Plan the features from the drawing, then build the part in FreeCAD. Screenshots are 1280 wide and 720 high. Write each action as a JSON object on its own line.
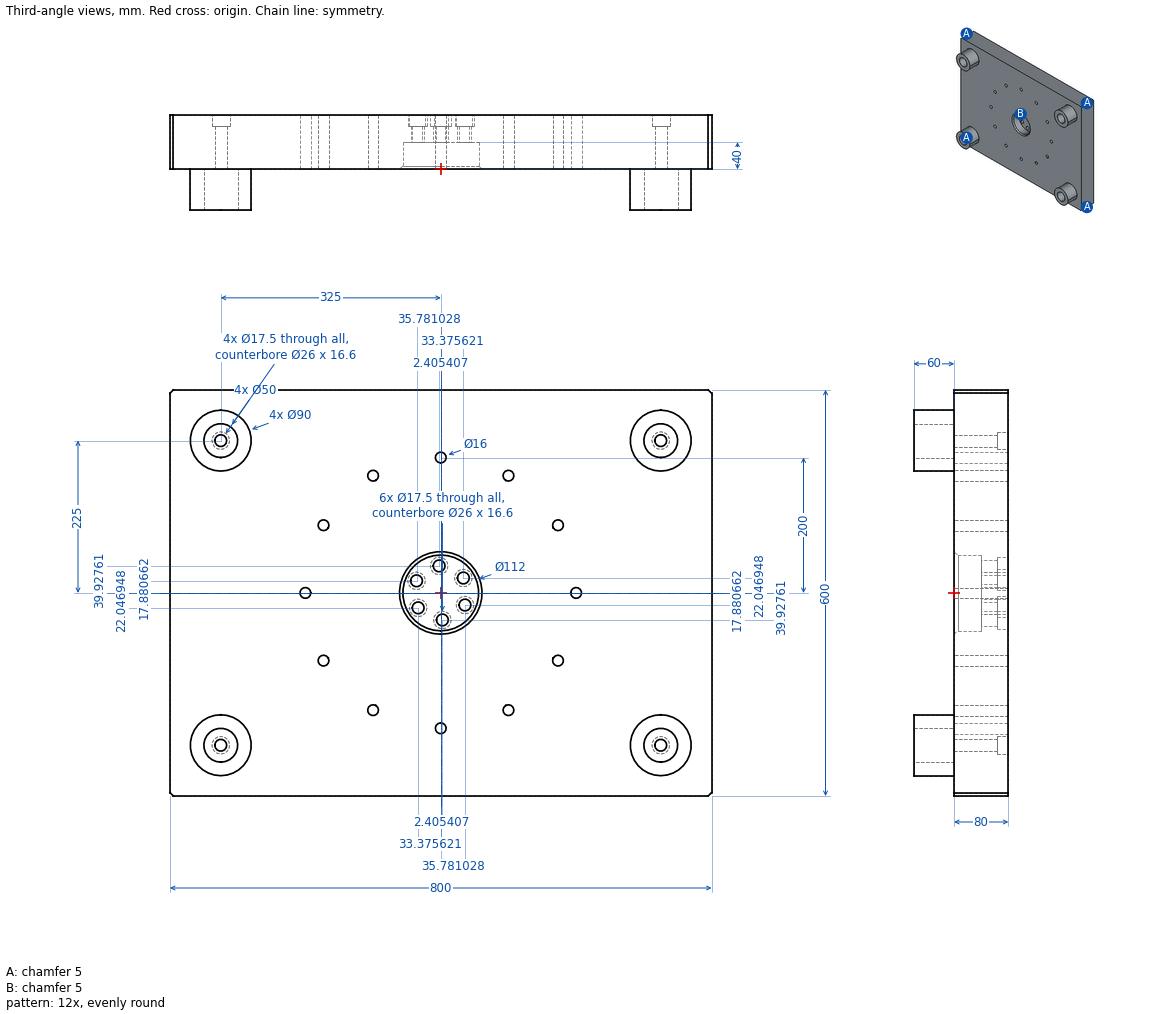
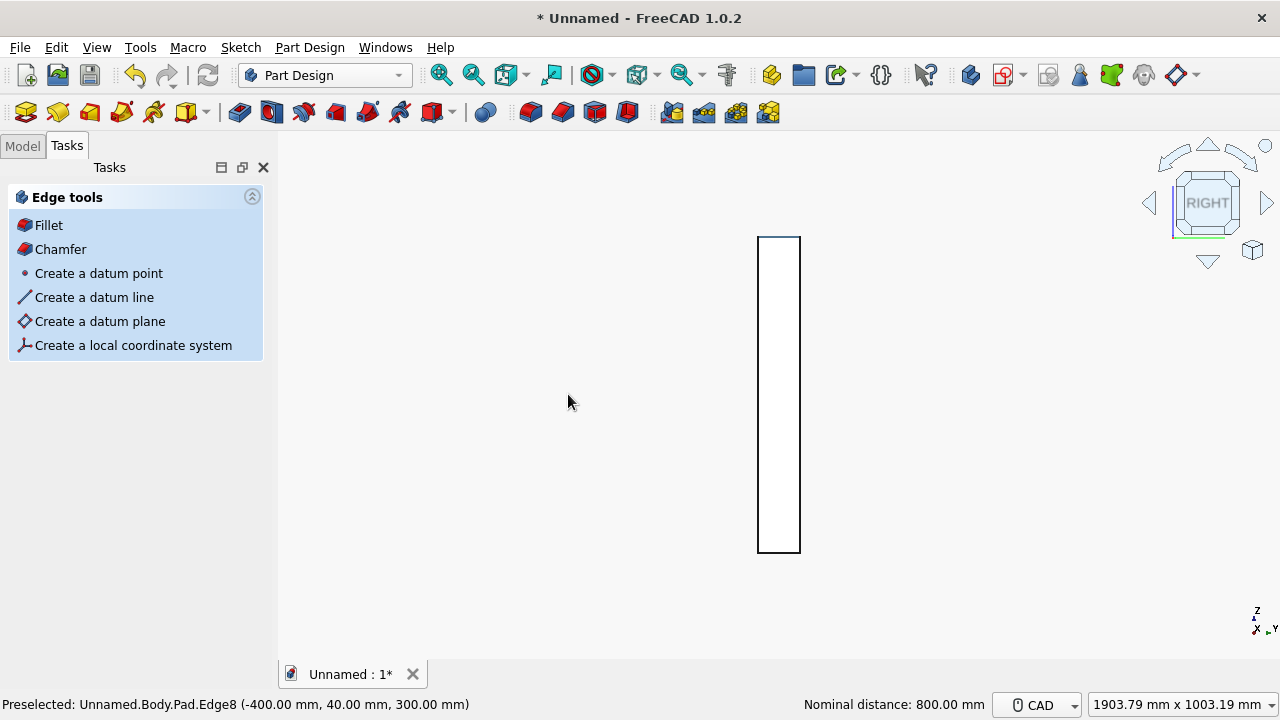
{"action": "left_click", "coordinate": [779, 552], "text": "ctrl"}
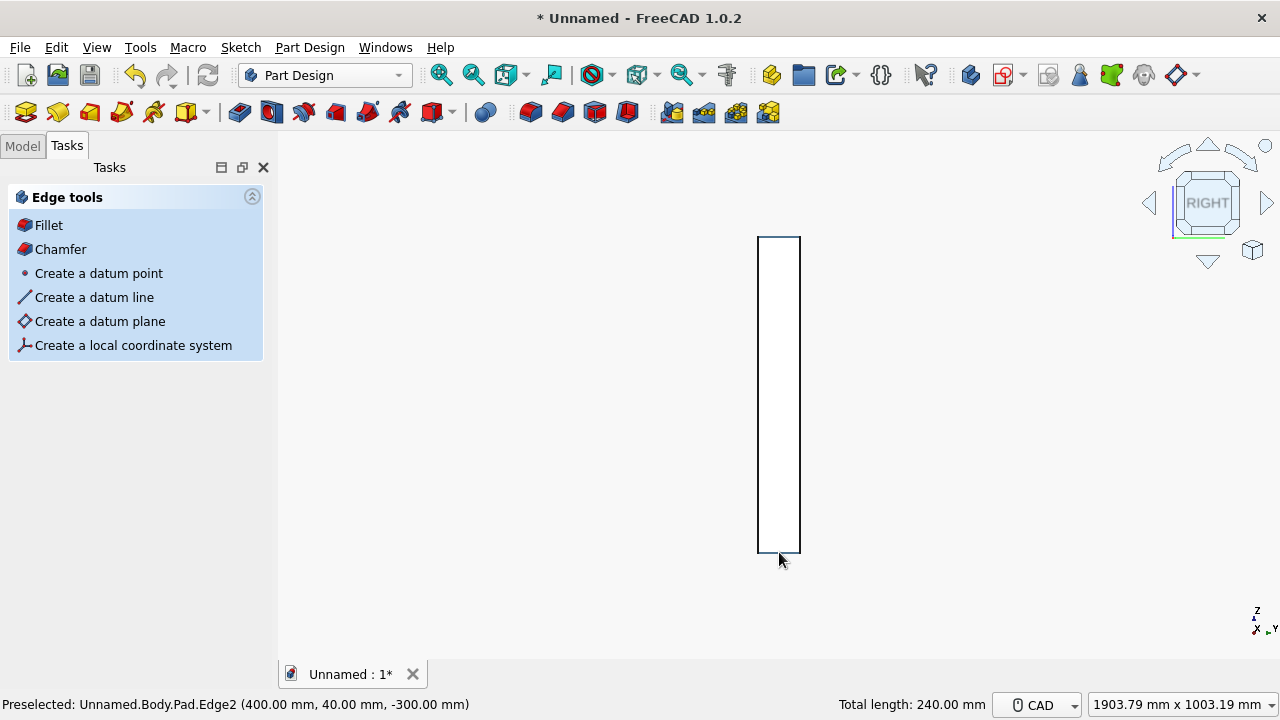
{"action": "key", "text": "5"}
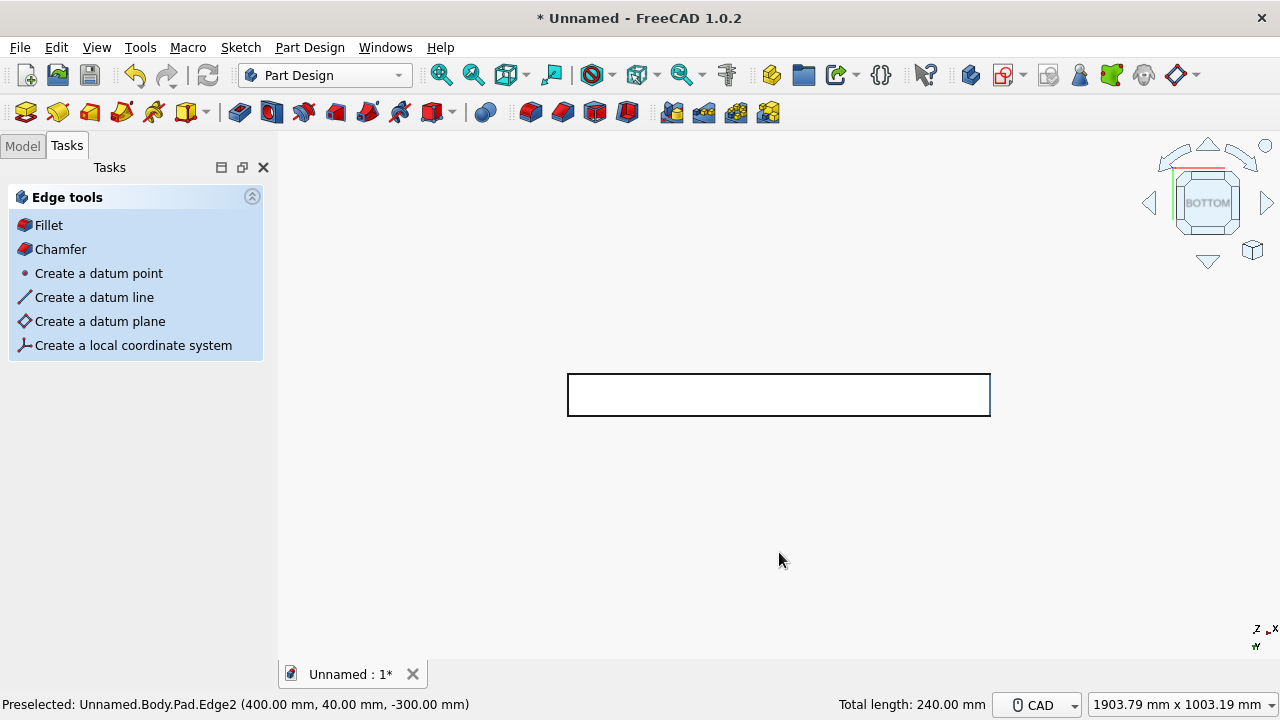
{"action": "left_click", "coordinate": [442, 76]}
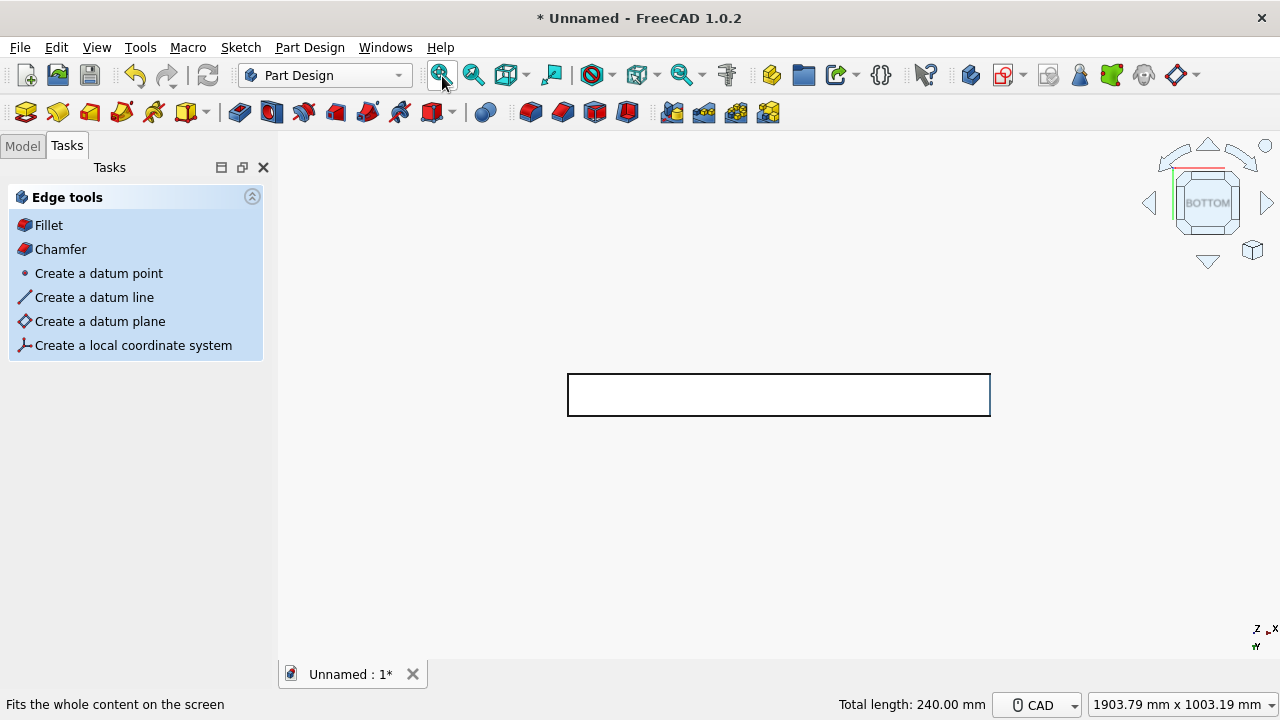
{"action": "left_click", "coordinate": [568, 394], "text": "ctrl"}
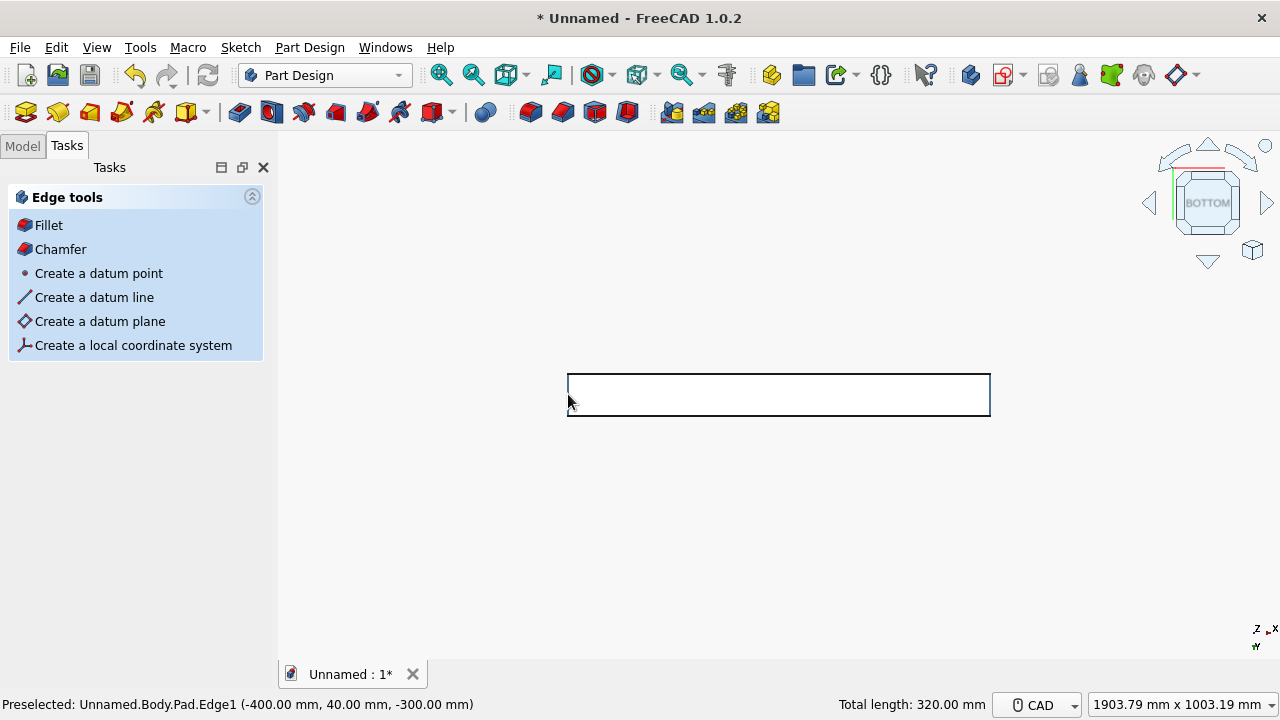
{"action": "left_click", "coordinate": [564, 112]}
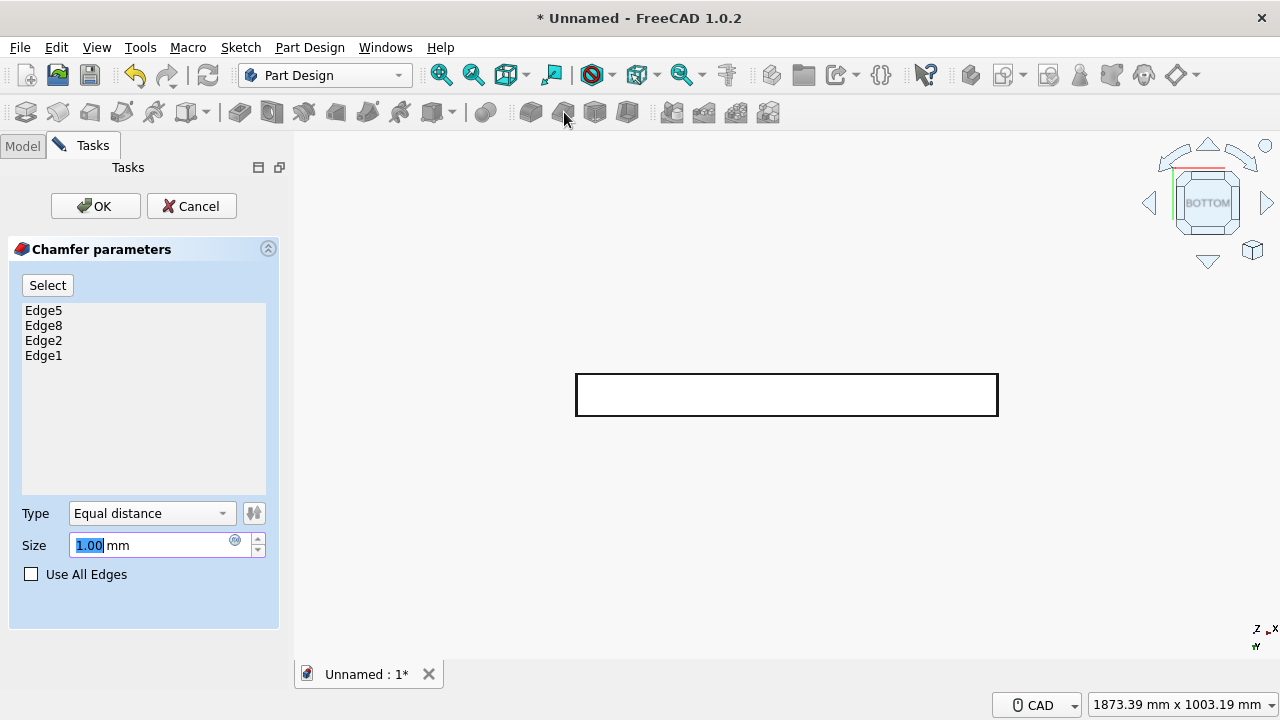
{"action": "type", "text": "5"}
{"action": "key", "text": "Tab"}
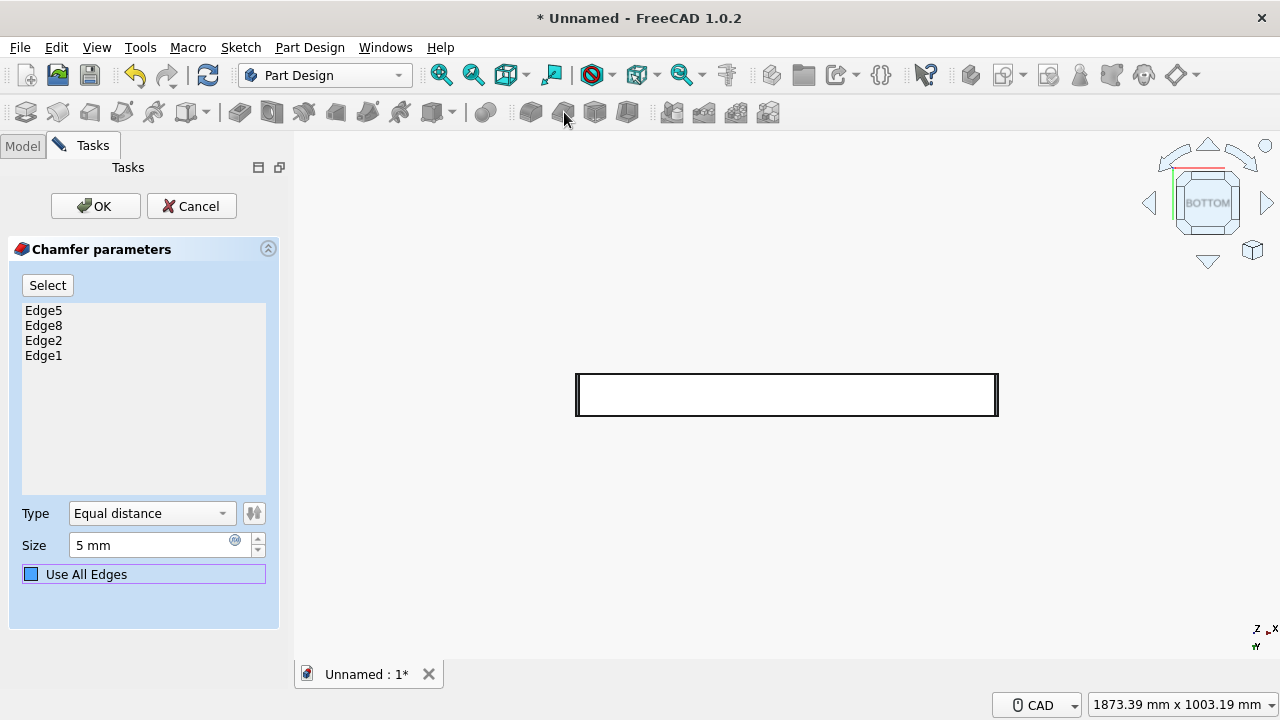
{"action": "left_click", "coordinate": [96, 206]}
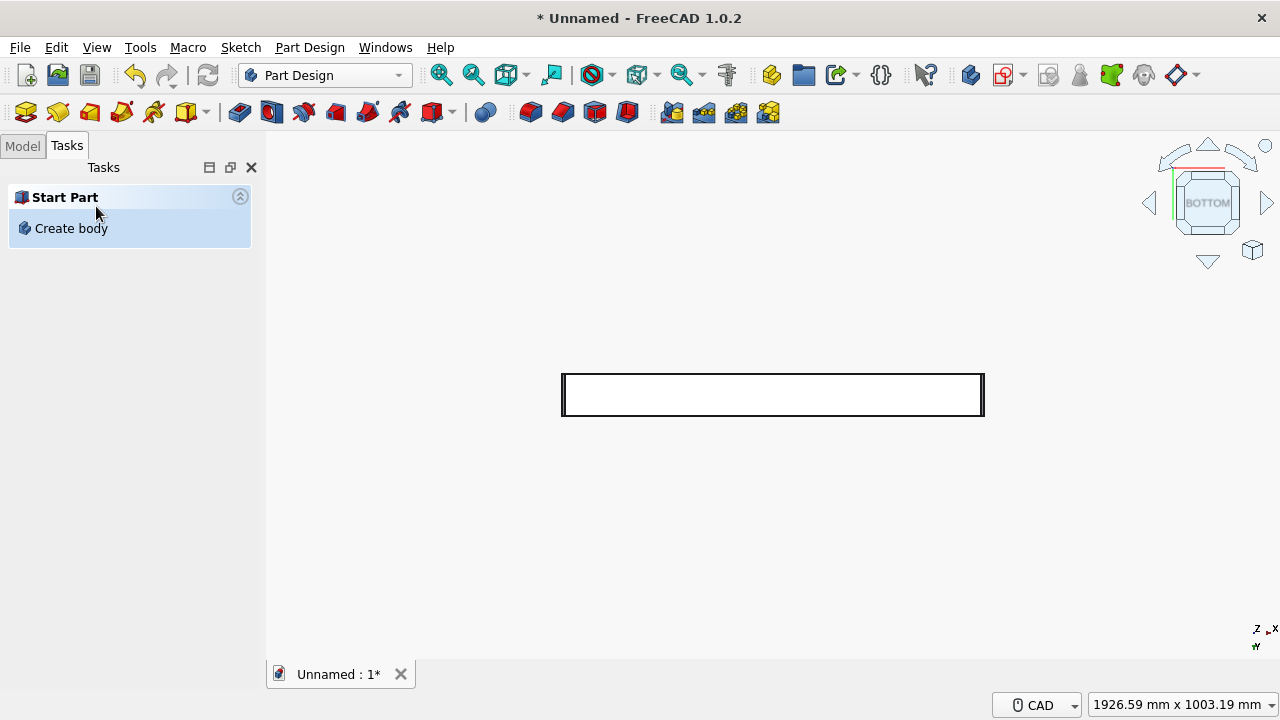
{"action": "left_click", "coordinate": [442, 76]}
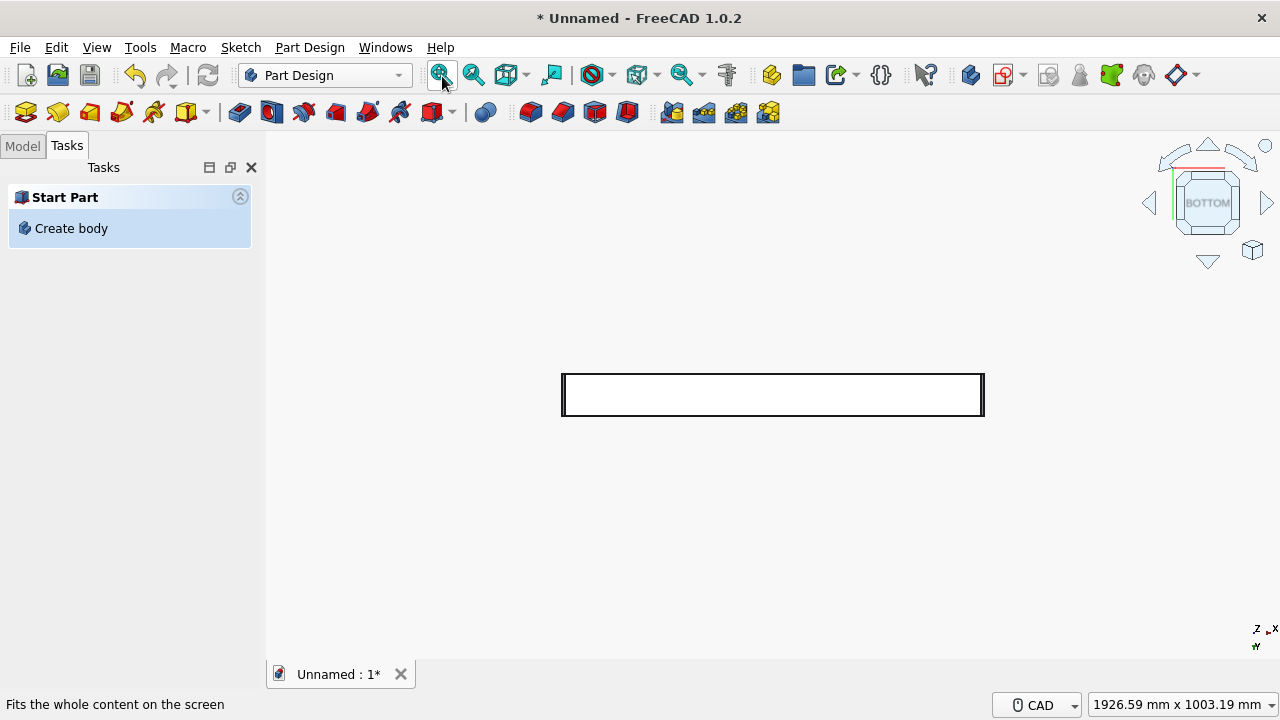
{"action": "key", "text": "4"}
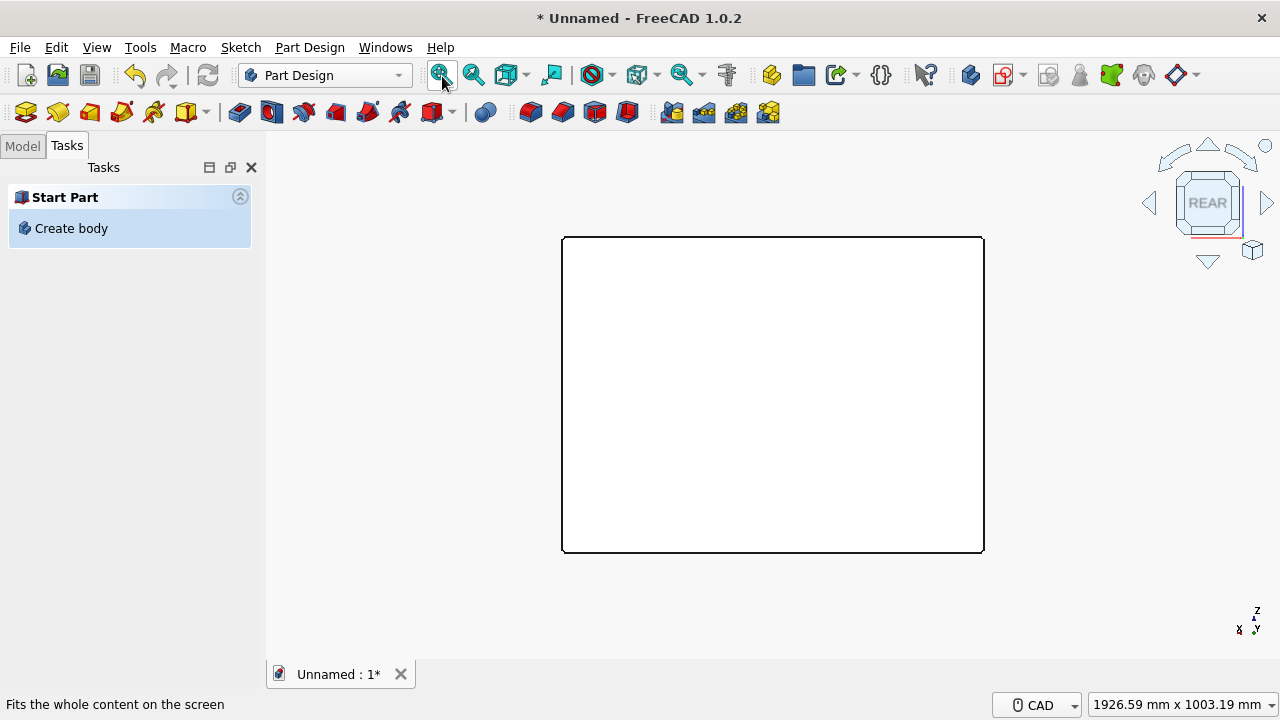
{"action": "left_click", "coordinate": [773, 394]}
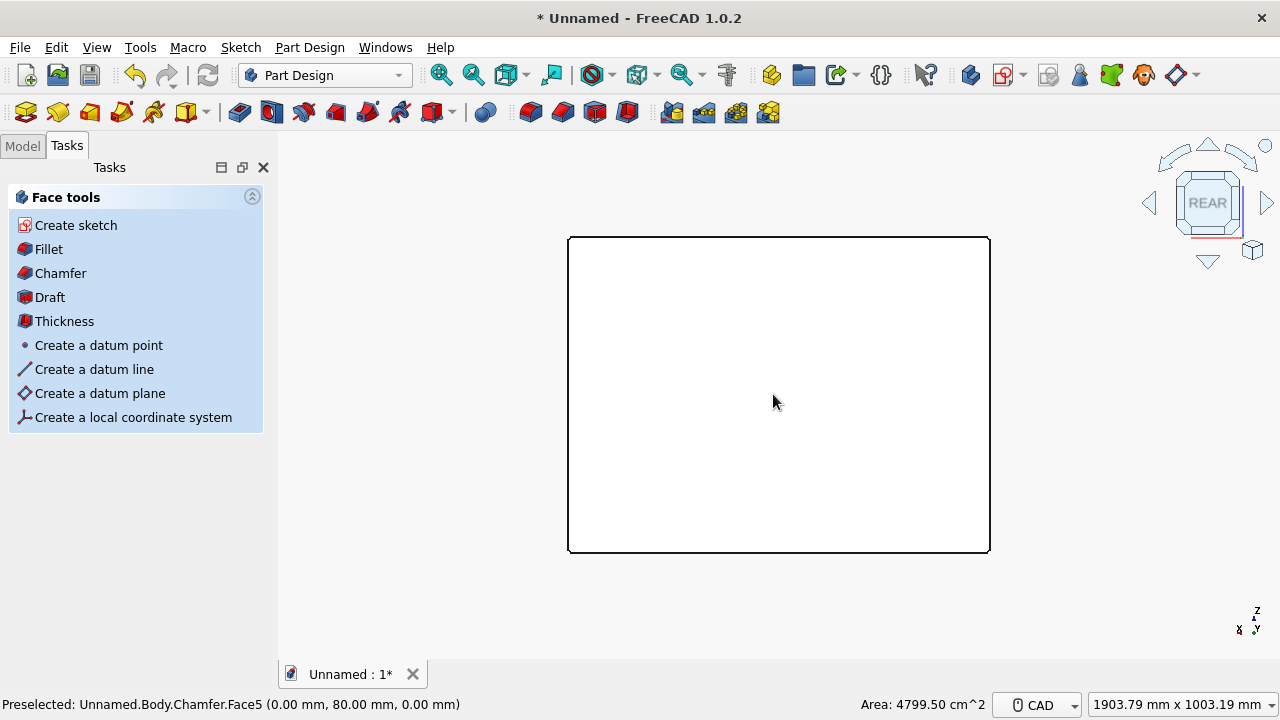
{"action": "left_click", "coordinate": [1004, 76]}